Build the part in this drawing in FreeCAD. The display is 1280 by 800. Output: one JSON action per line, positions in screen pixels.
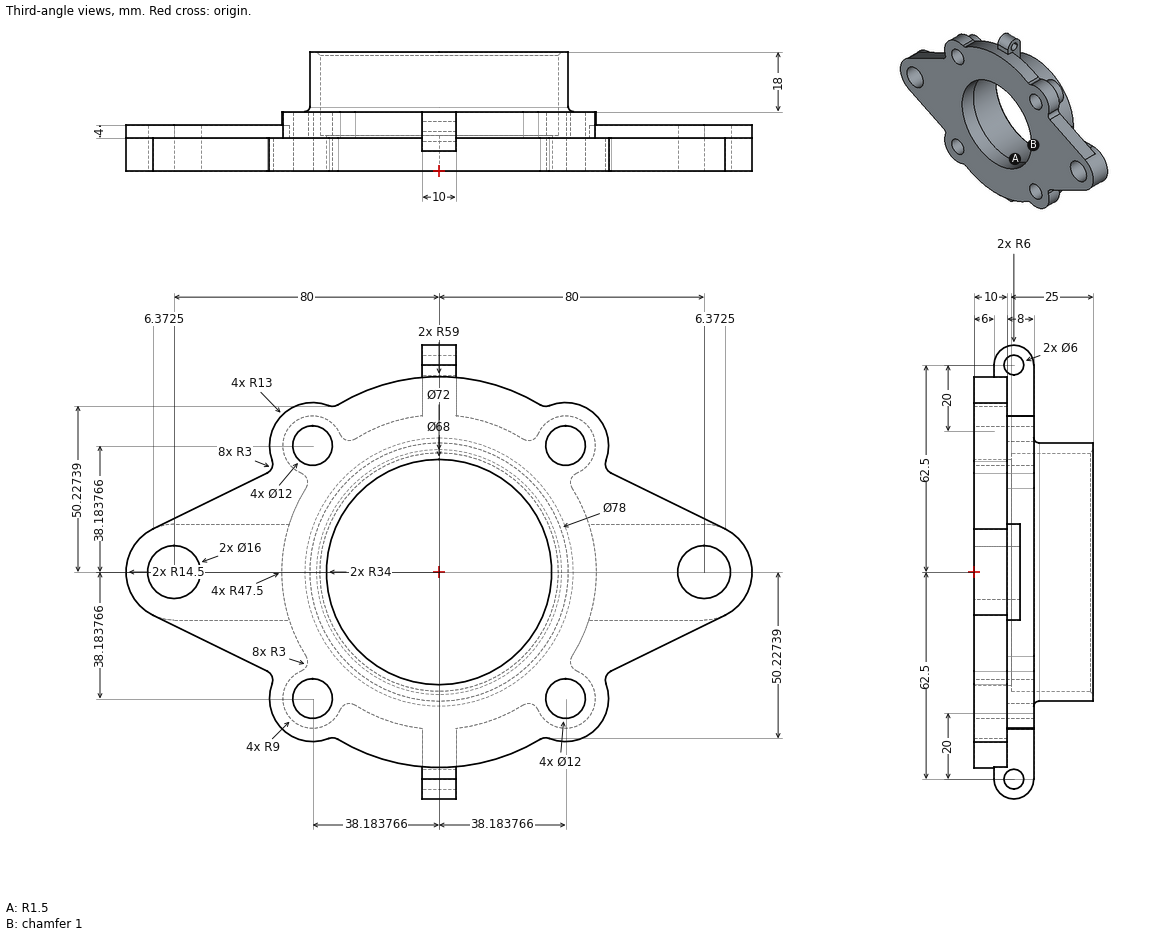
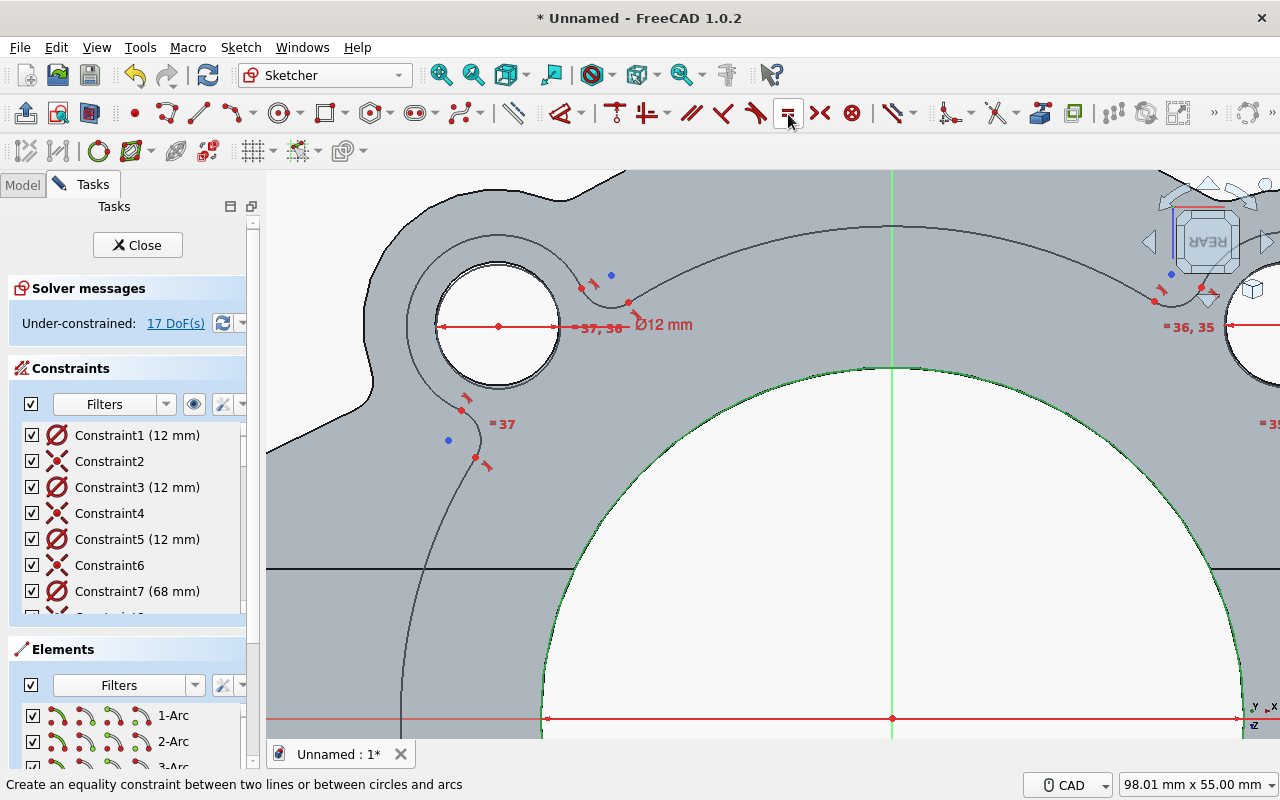
{"action": "left_click", "coordinate": [413, 610]}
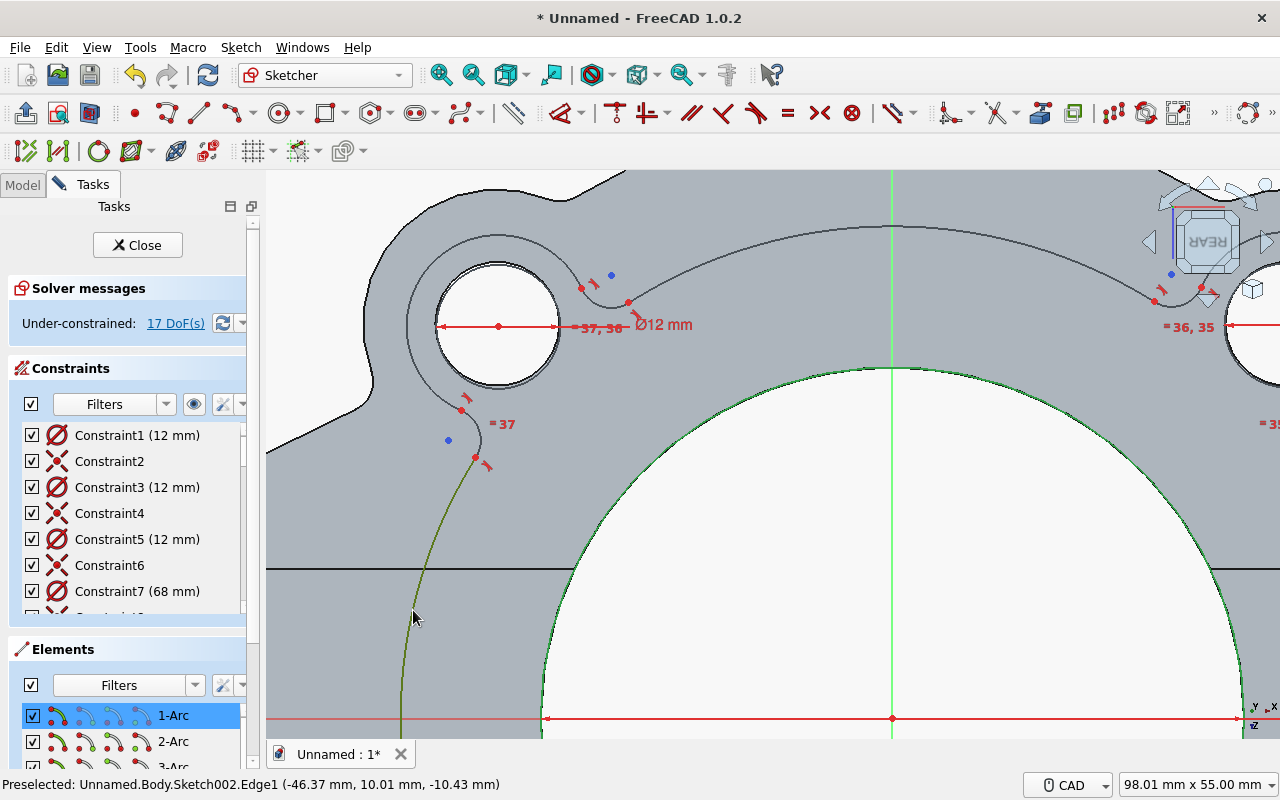
{"action": "scroll", "coordinate": [595, 301], "scroll_direction": "down", "scroll_amount": 5}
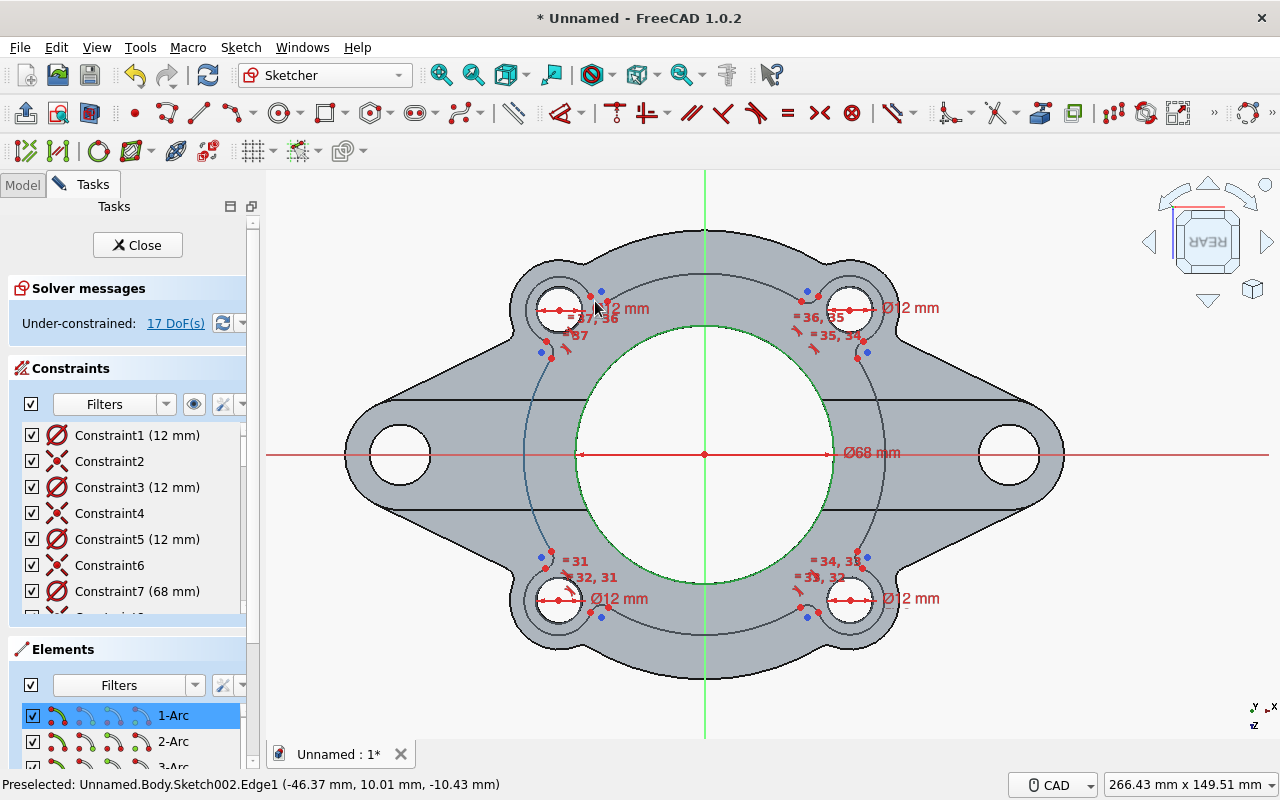
{"action": "left_click", "coordinate": [664, 630]}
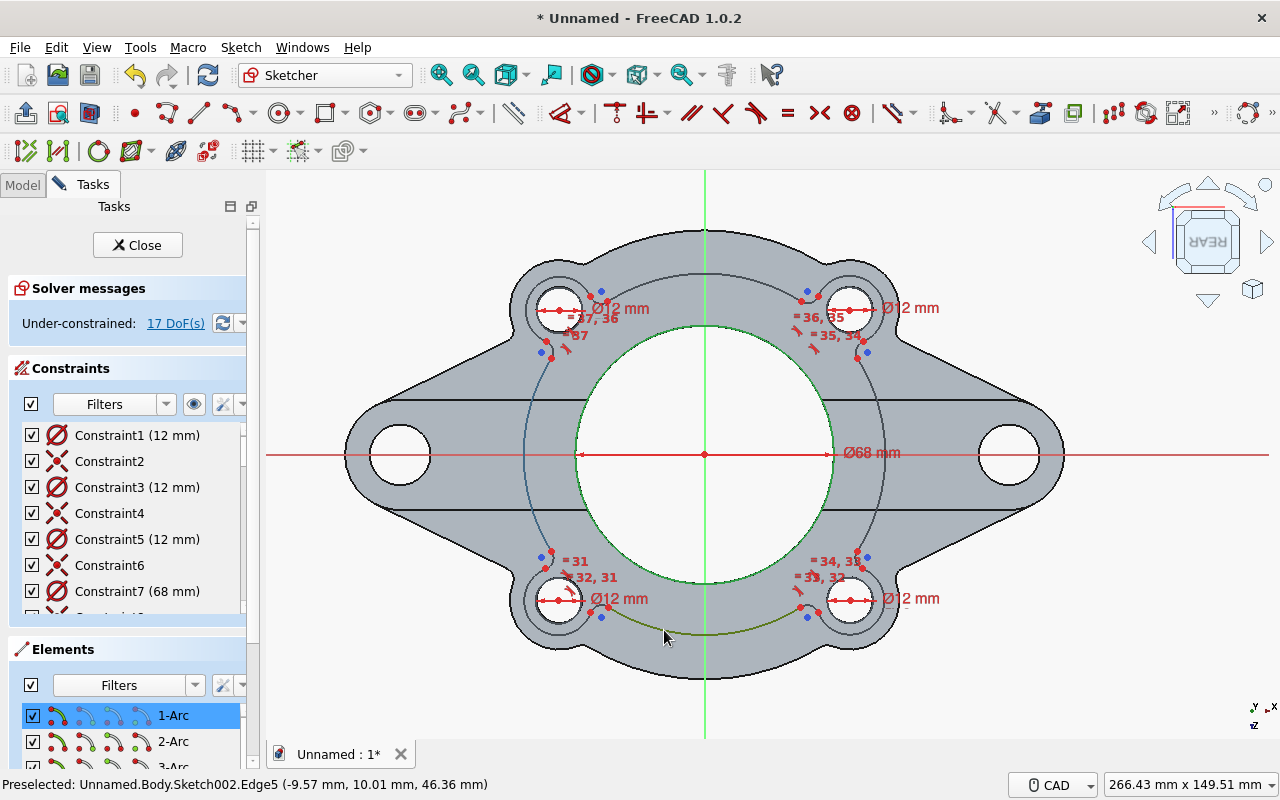
{"action": "left_click", "coordinate": [881, 496]}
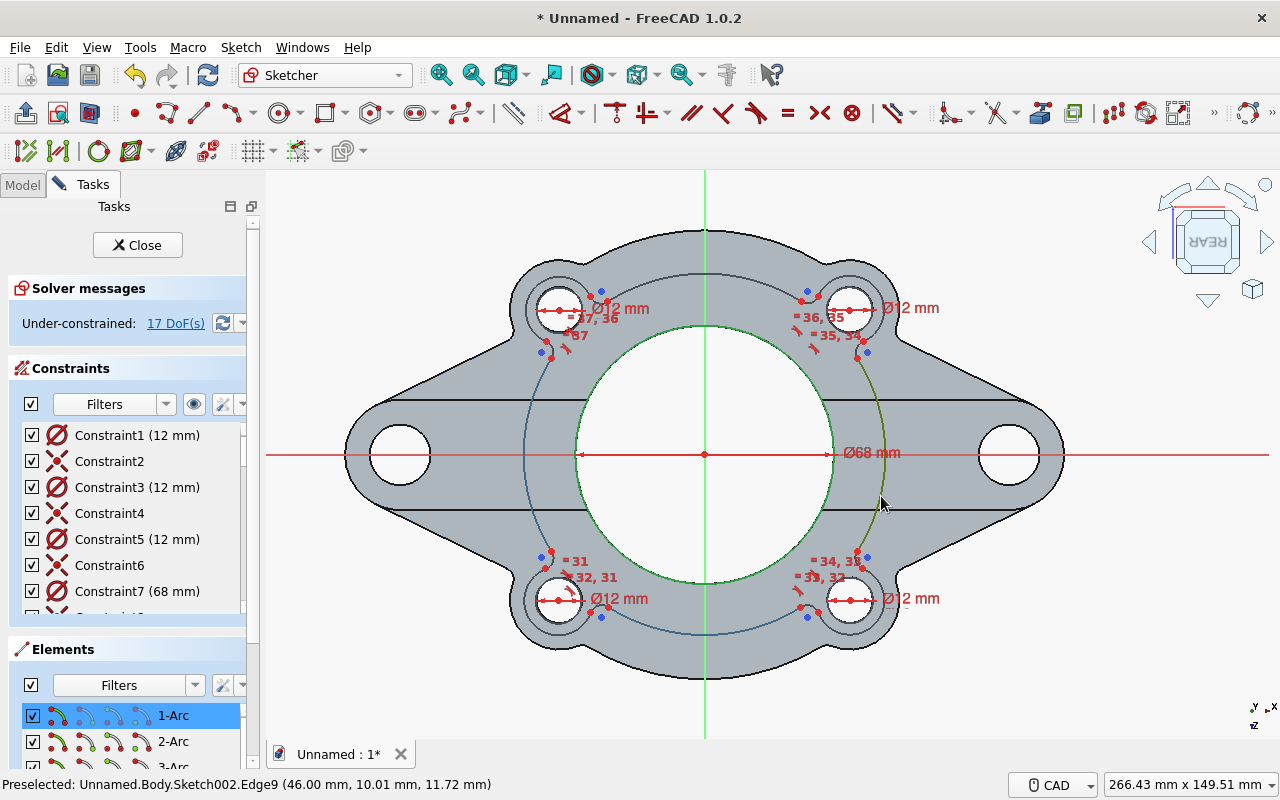
{"action": "left_click", "coordinate": [745, 278]}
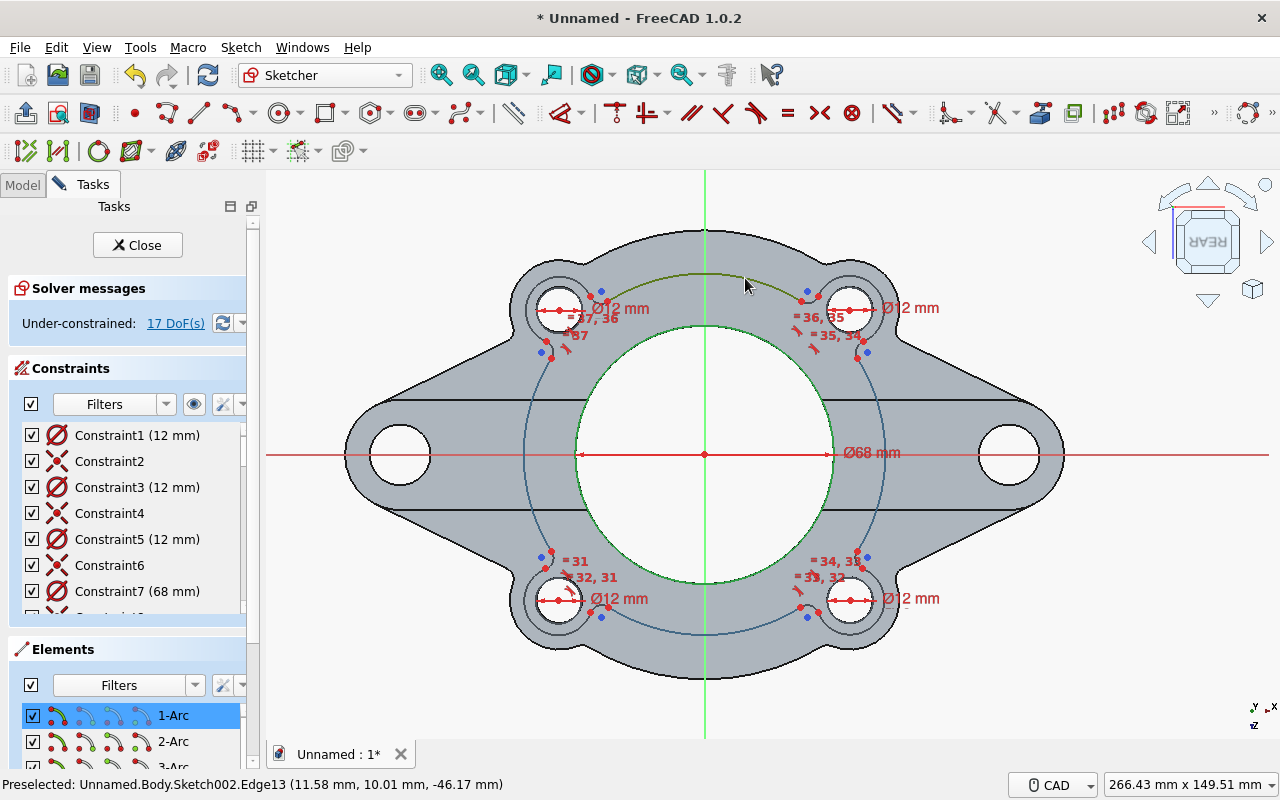
{"action": "left_click", "coordinate": [788, 114]}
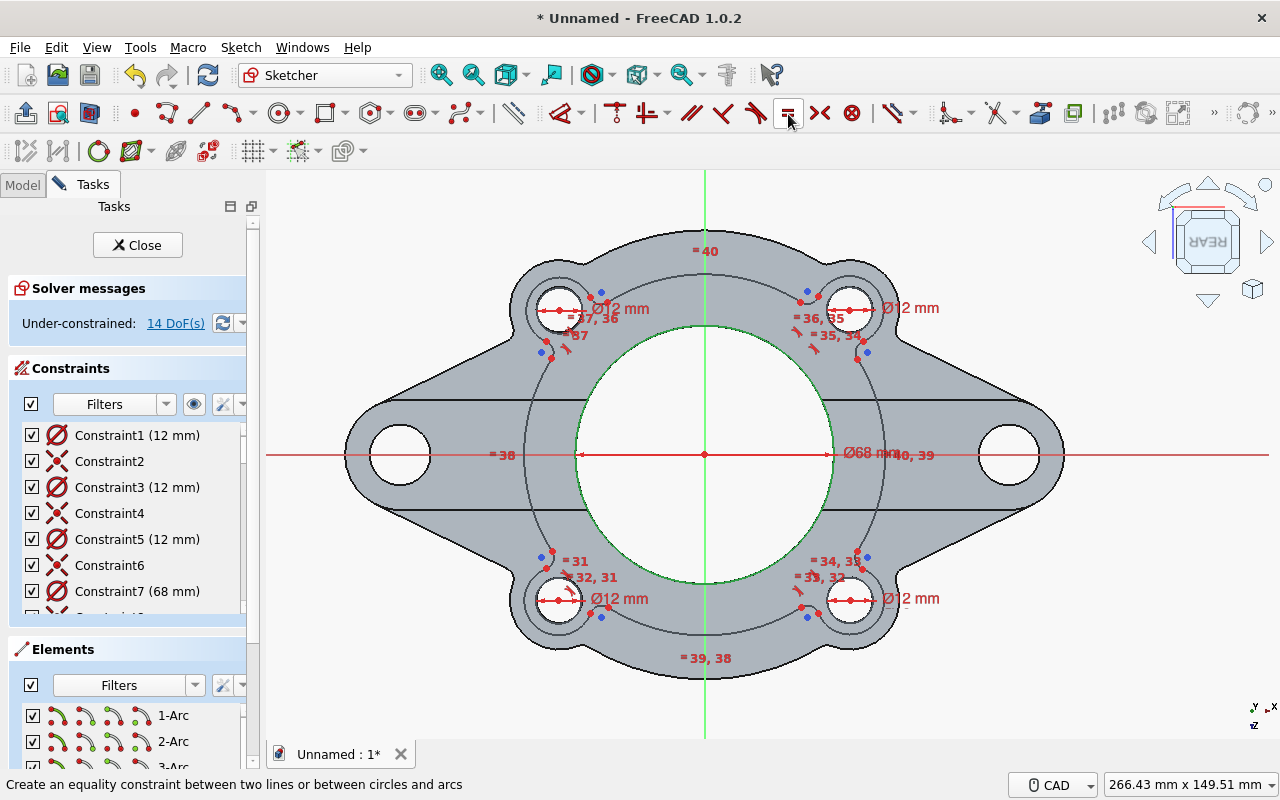
{"action": "left_click", "coordinate": [524, 601]}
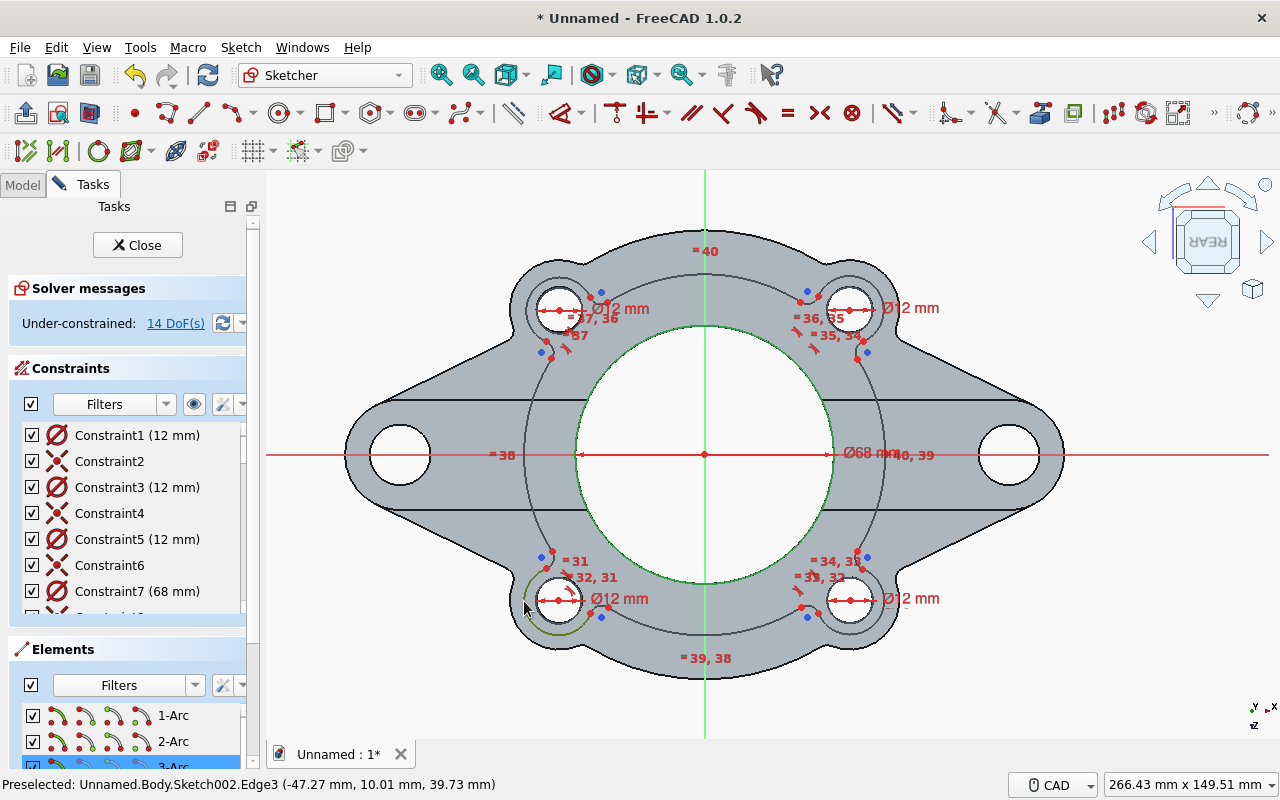
{"action": "scroll", "coordinate": [850, 635], "scroll_direction": "up", "scroll_amount": 2}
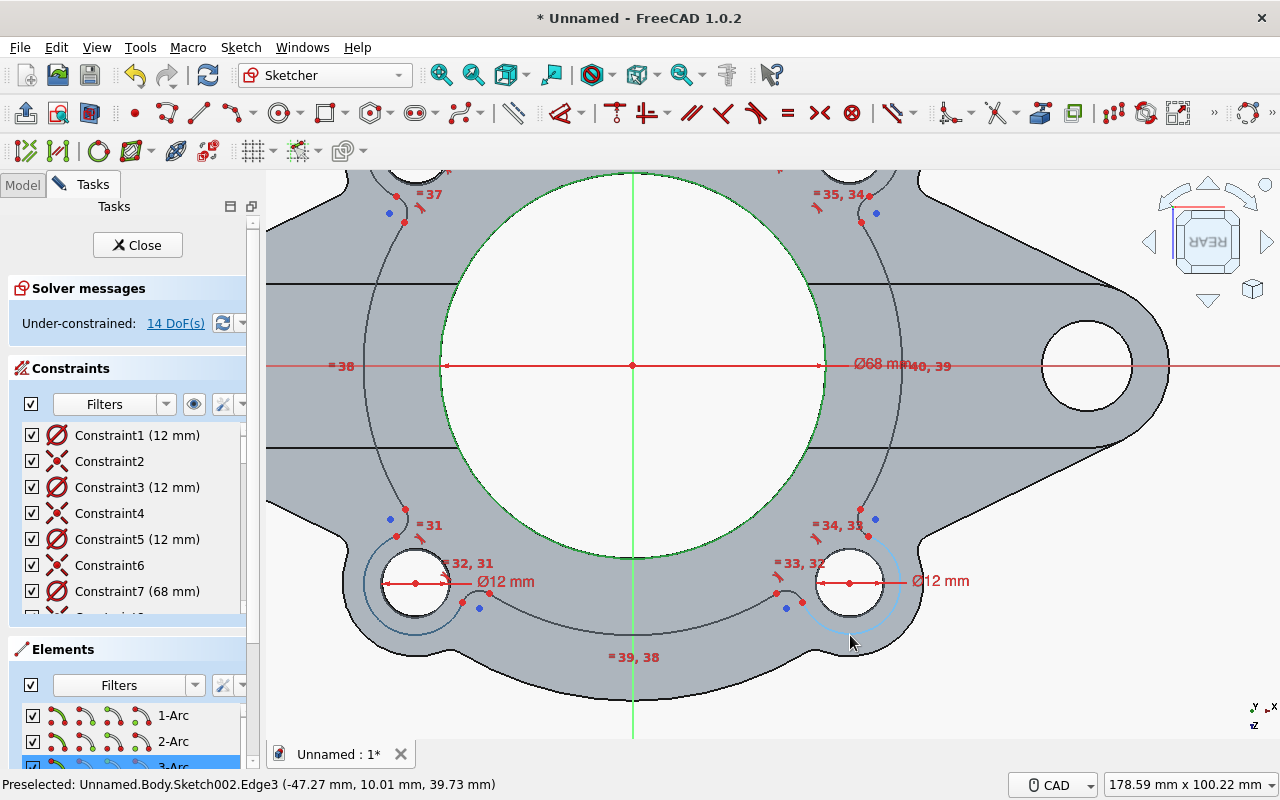
{"action": "left_click", "coordinate": [850, 634]}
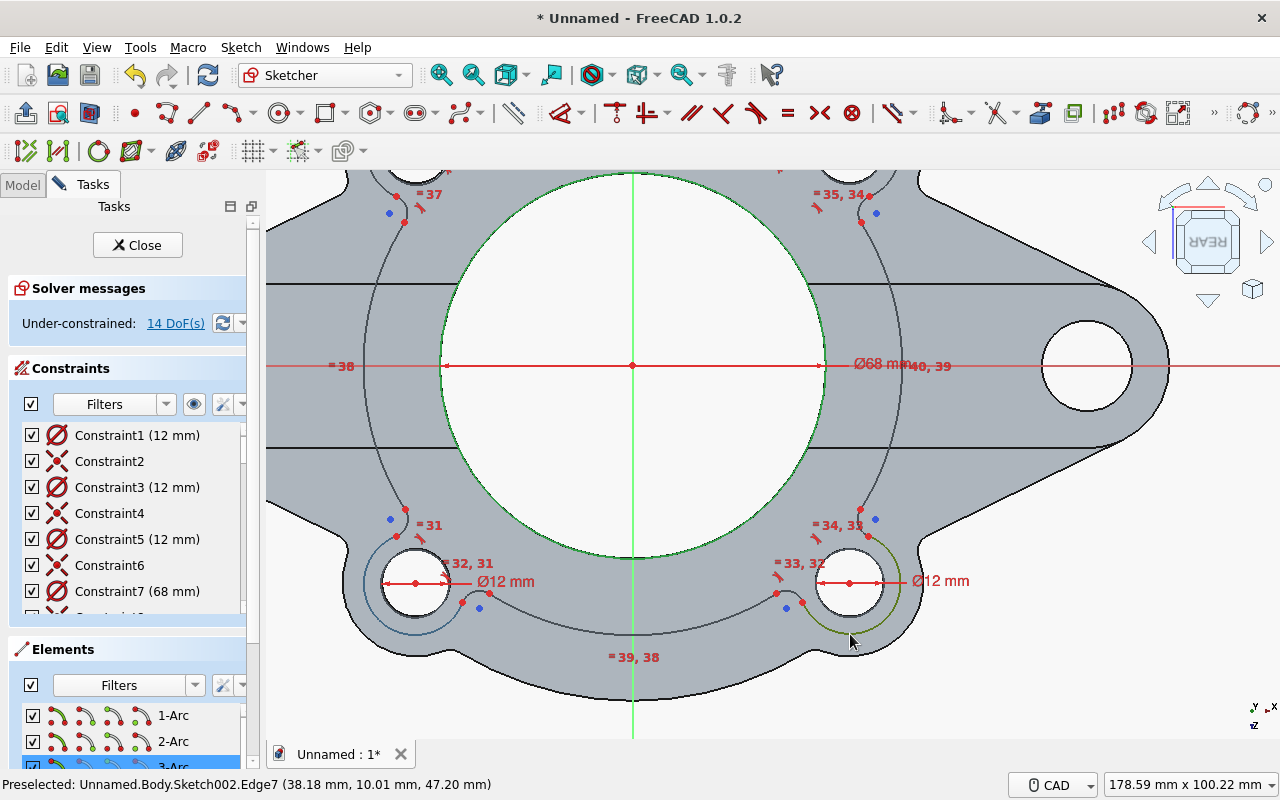
{"action": "scroll", "coordinate": [850, 635], "scroll_direction": "down", "scroll_amount": 2}